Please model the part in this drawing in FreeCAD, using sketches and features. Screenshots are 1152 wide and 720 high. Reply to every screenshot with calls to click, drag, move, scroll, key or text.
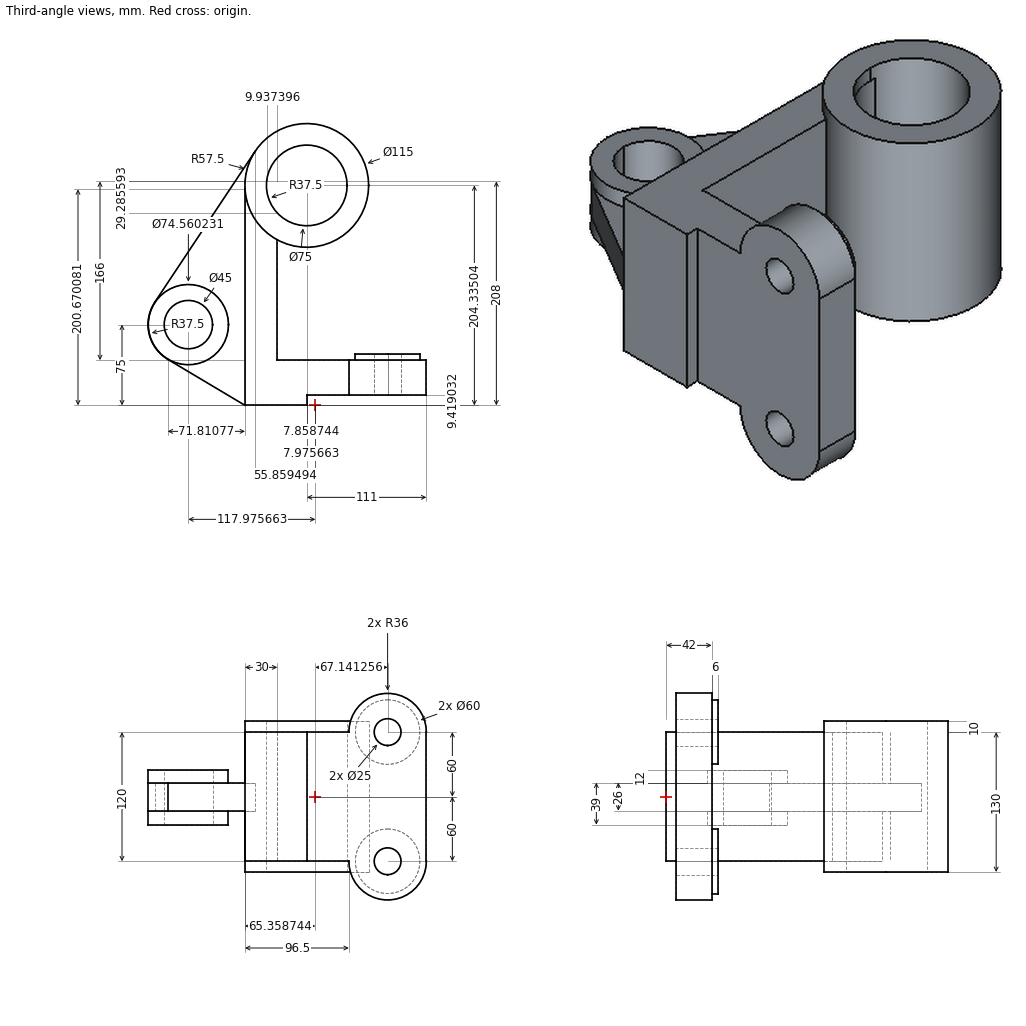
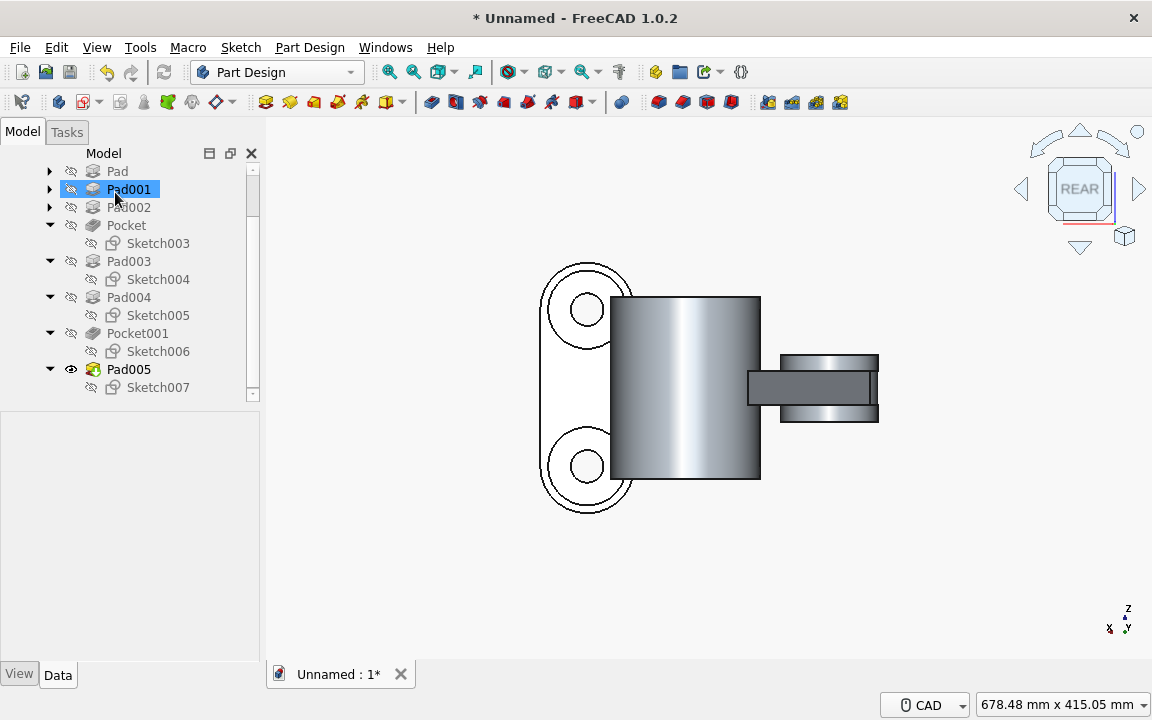
key(0)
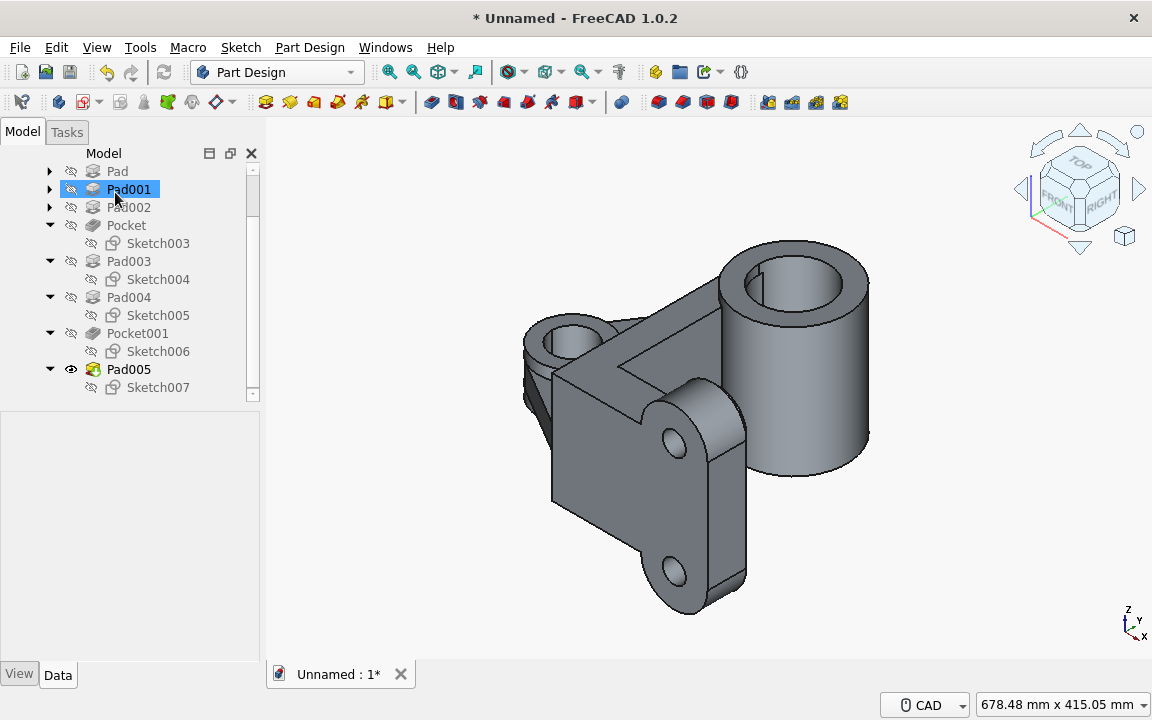
click(635, 405)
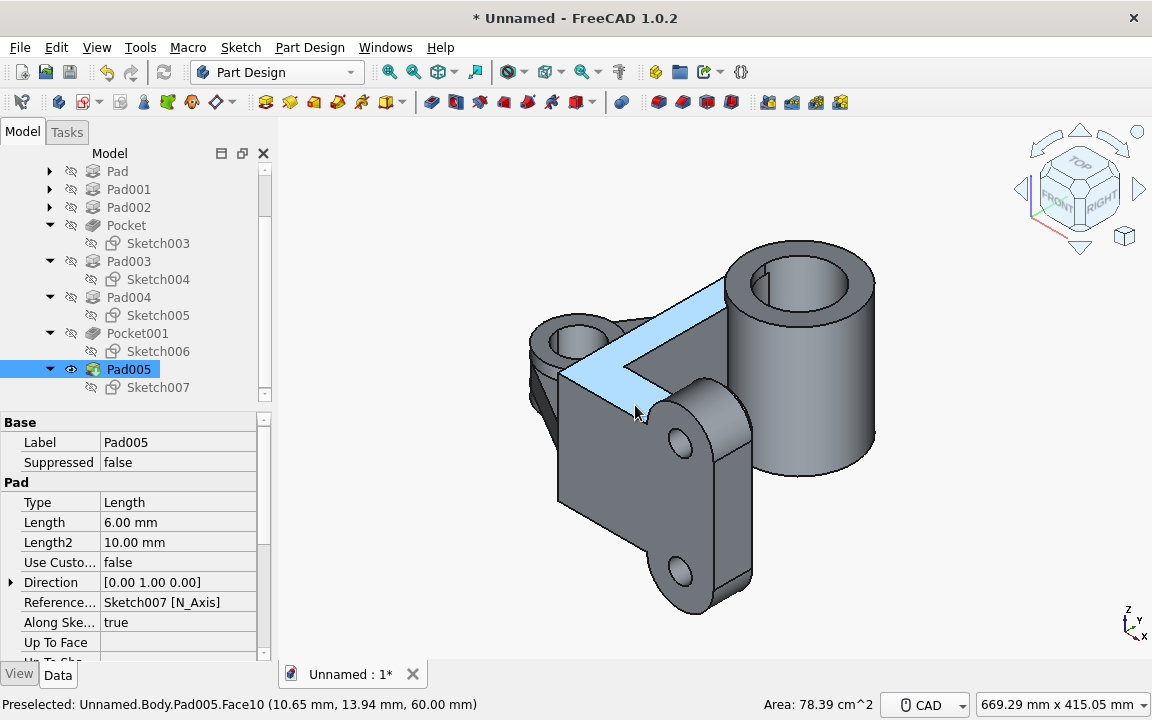
click(84, 102)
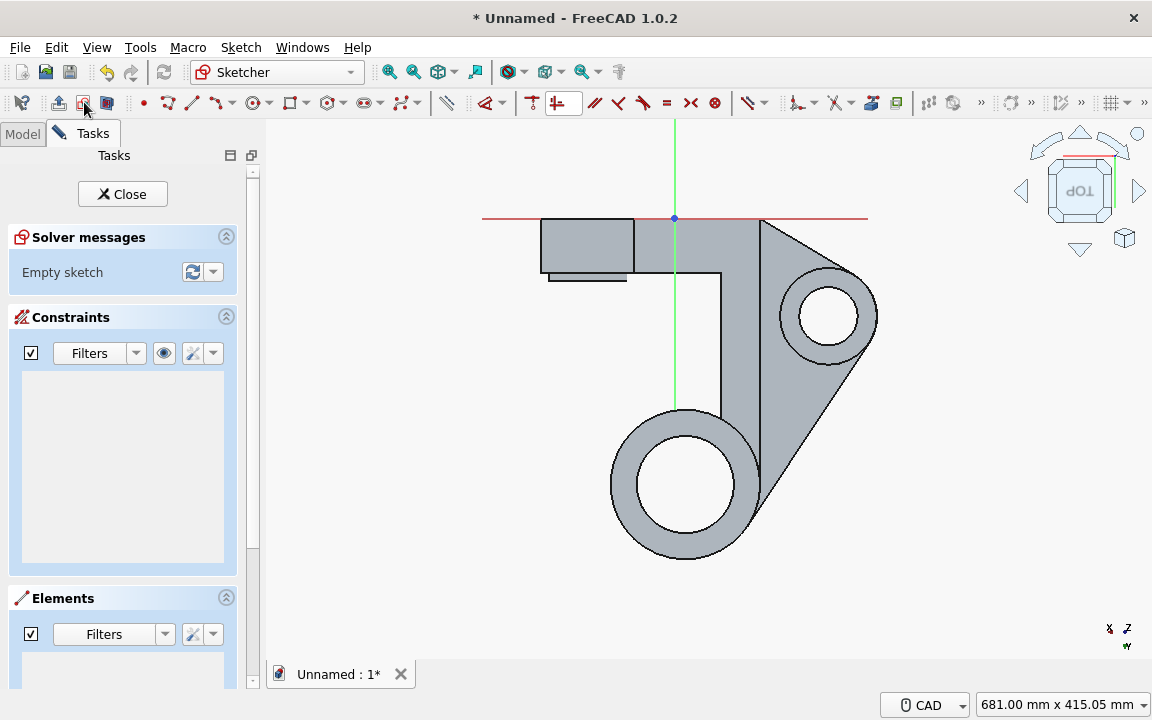
scroll(601, 154, up, 6)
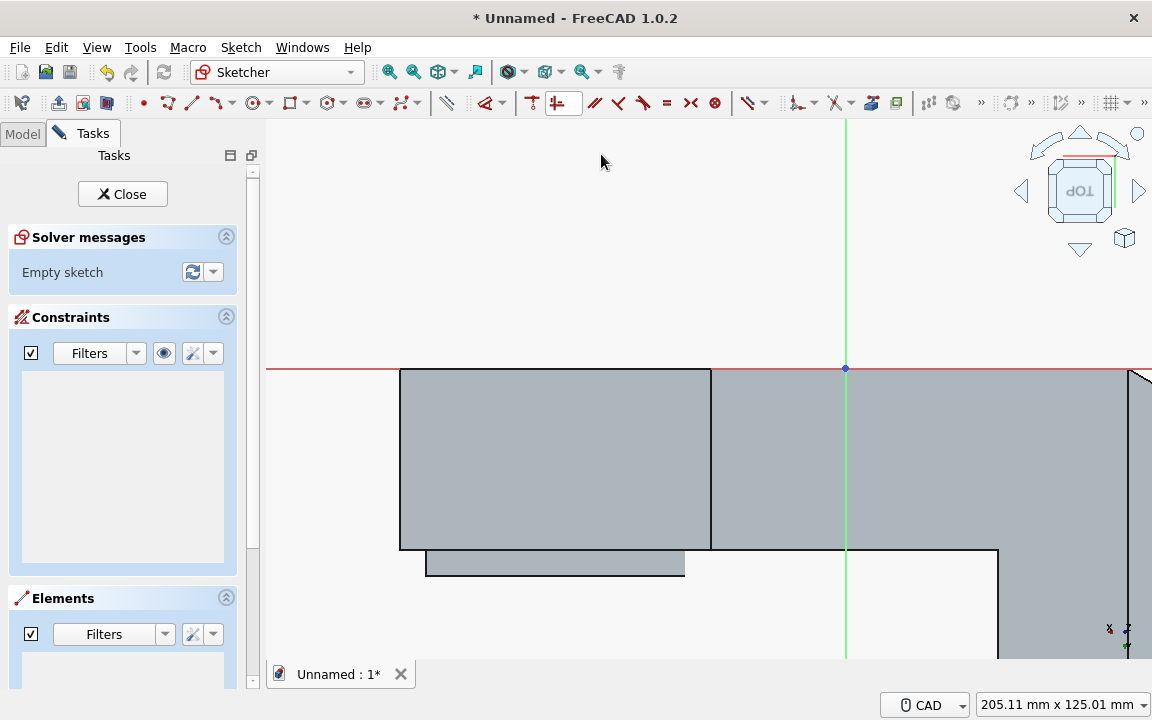
click(290, 104)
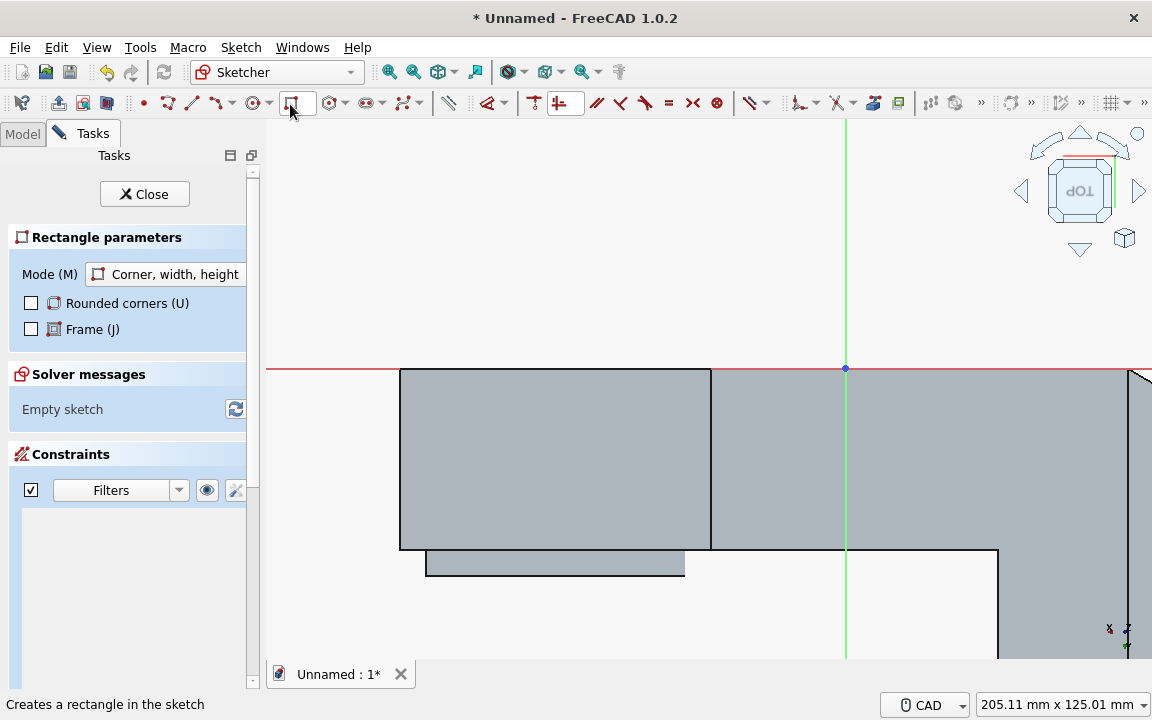
click(400, 369)
move(880, 409)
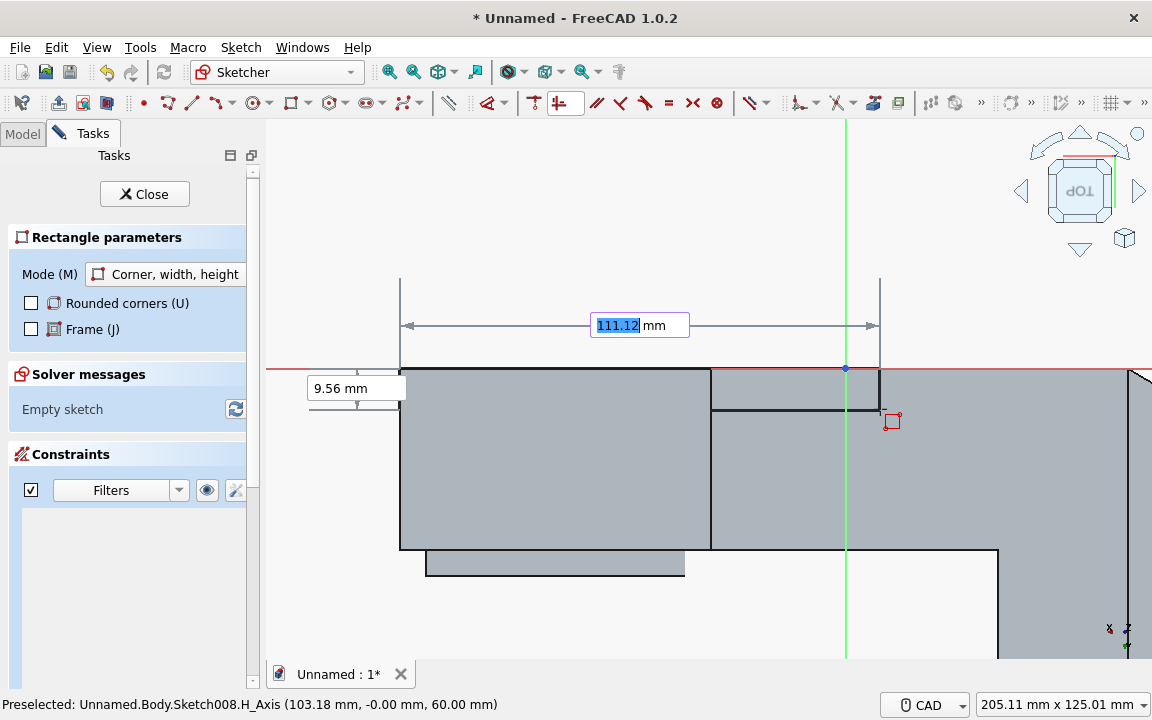
text(111)
key(Tab)
text(9.419032)
key(Return)
key(Escape)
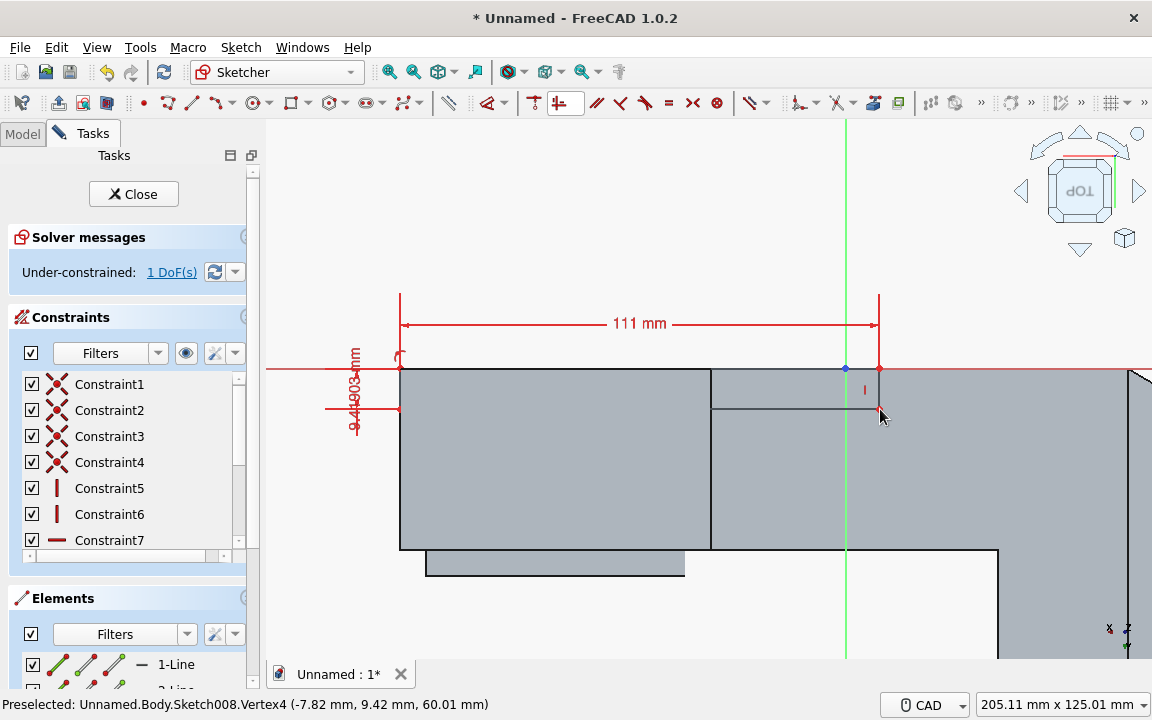
click(488, 104)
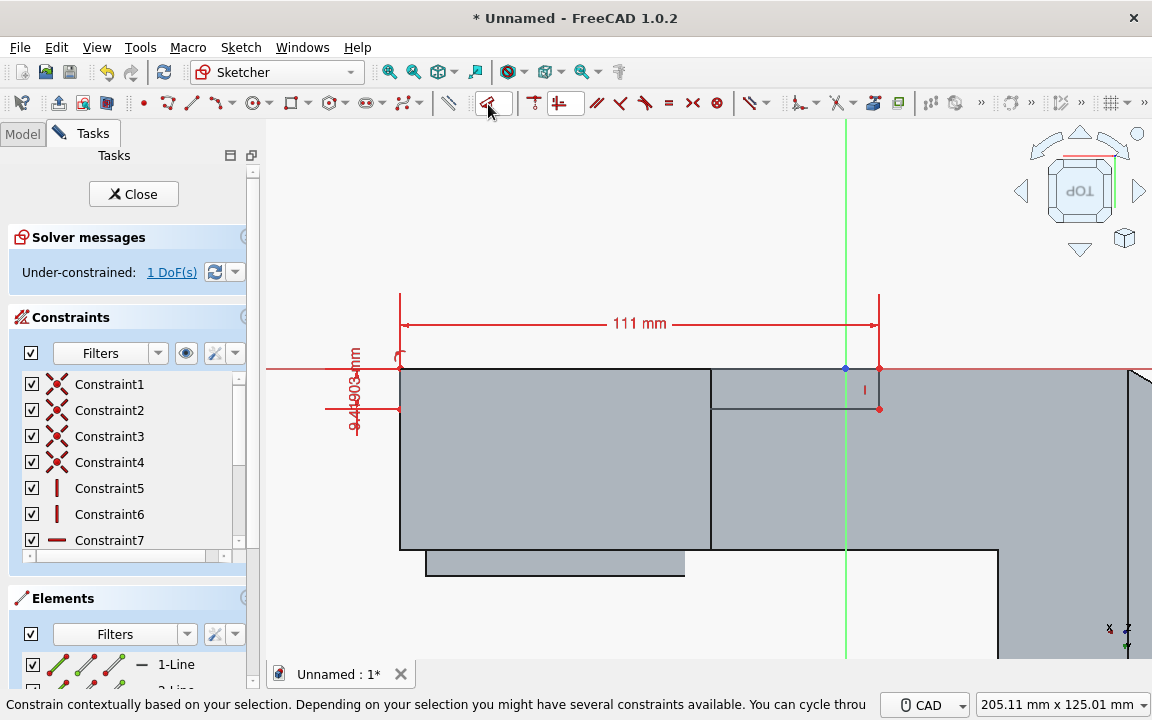
click(879, 409)
click(863, 443)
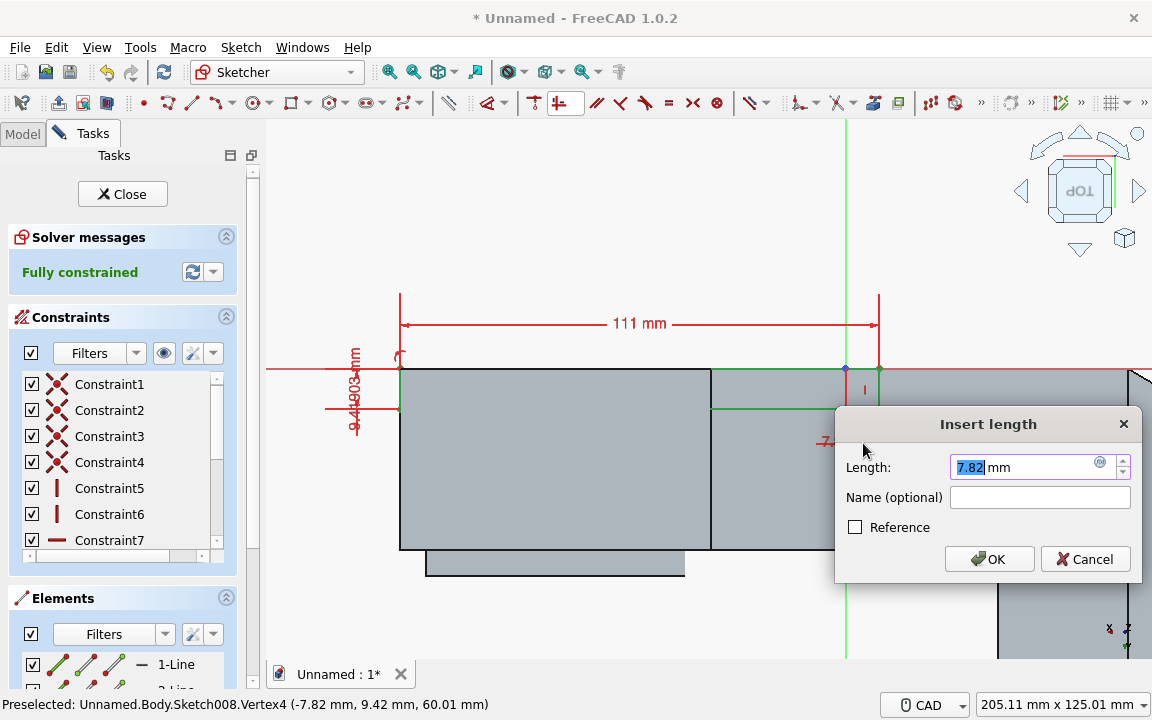
text(7.858744)
key(Return)
key(Escape)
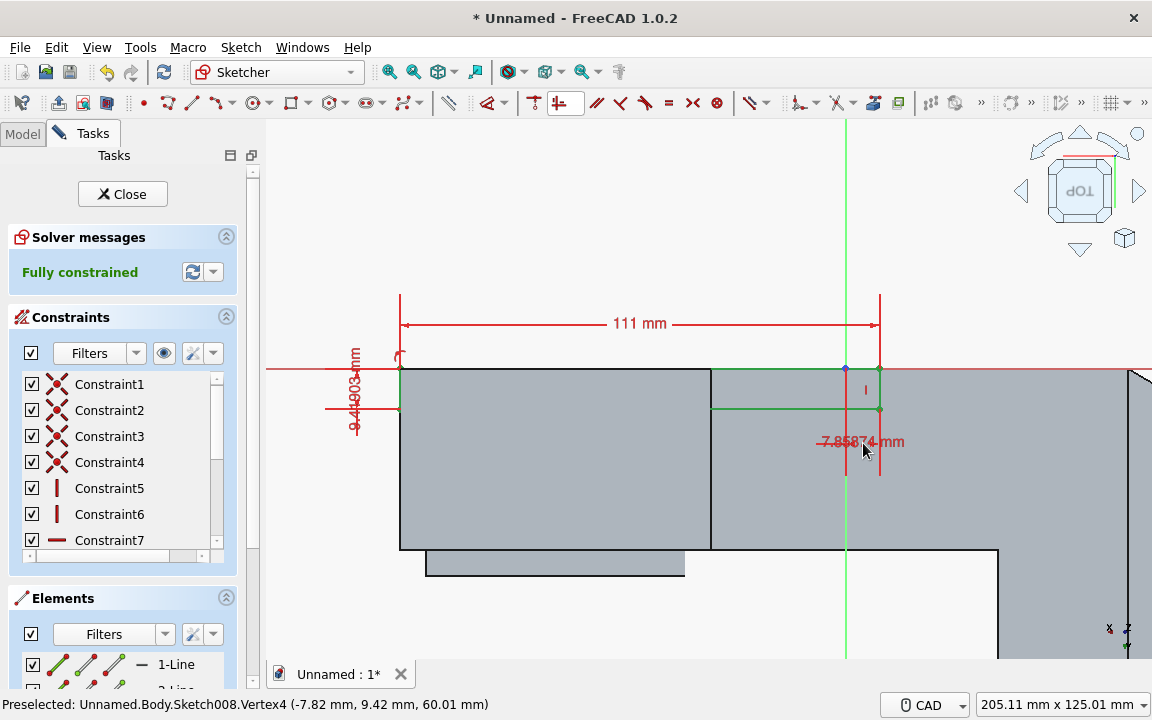
click(123, 194)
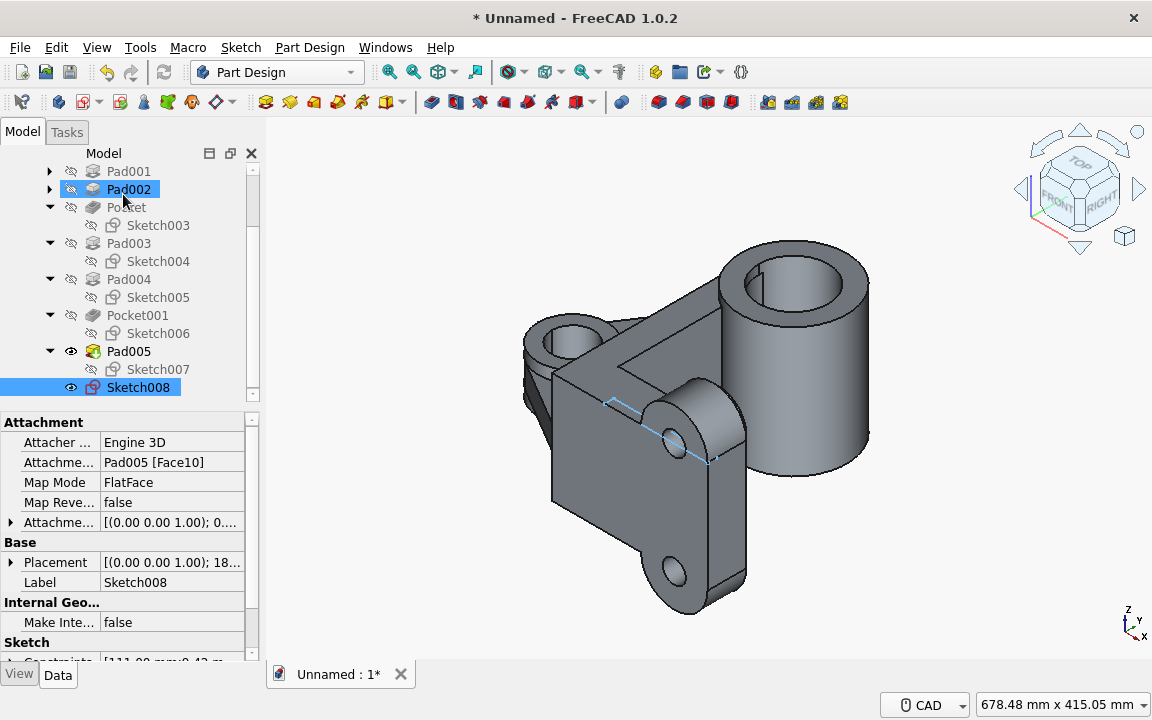
click(432, 102)